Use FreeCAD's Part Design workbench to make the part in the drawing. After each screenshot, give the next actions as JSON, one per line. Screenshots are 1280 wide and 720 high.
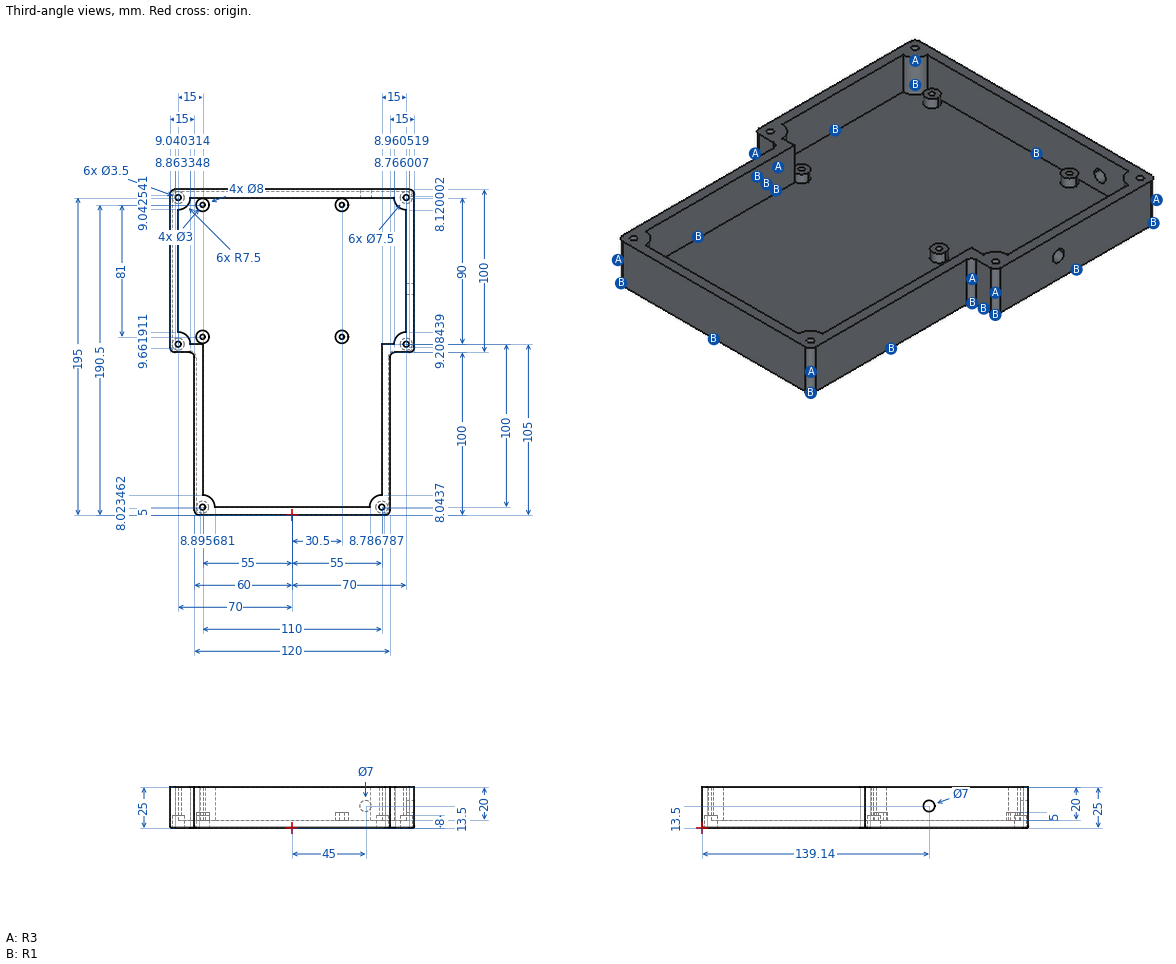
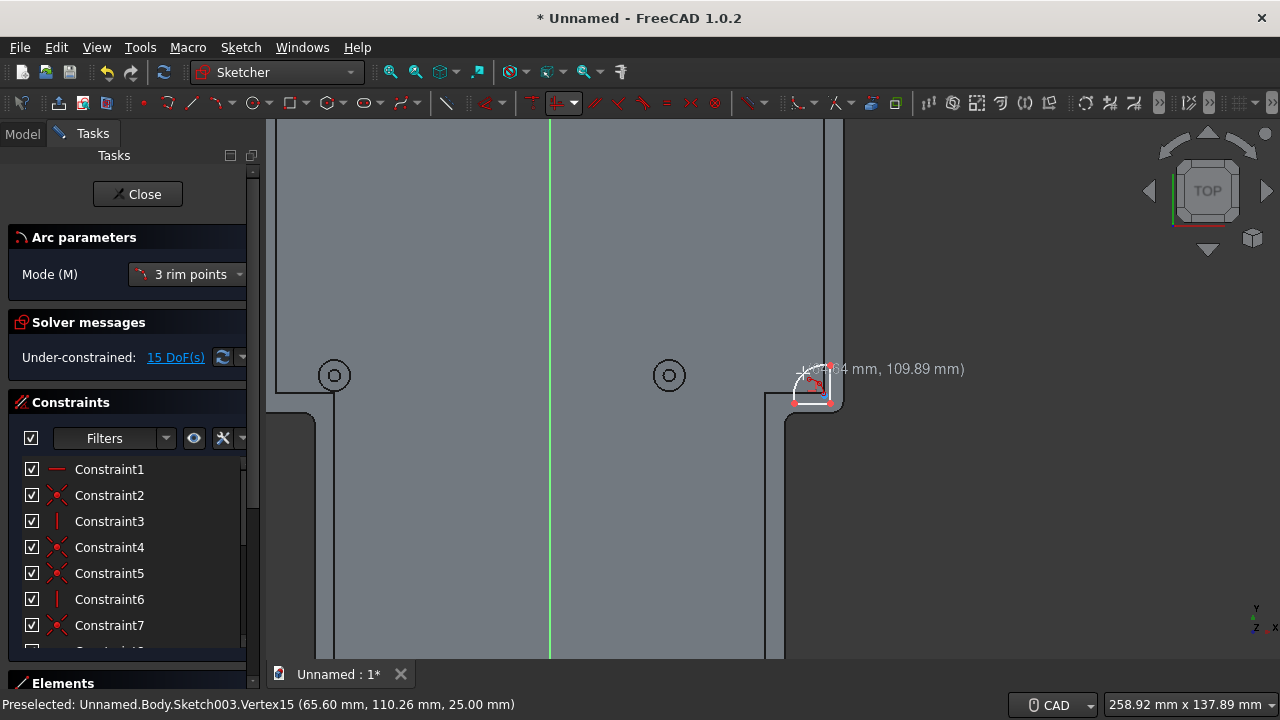
{"action": "key", "text": "g m"}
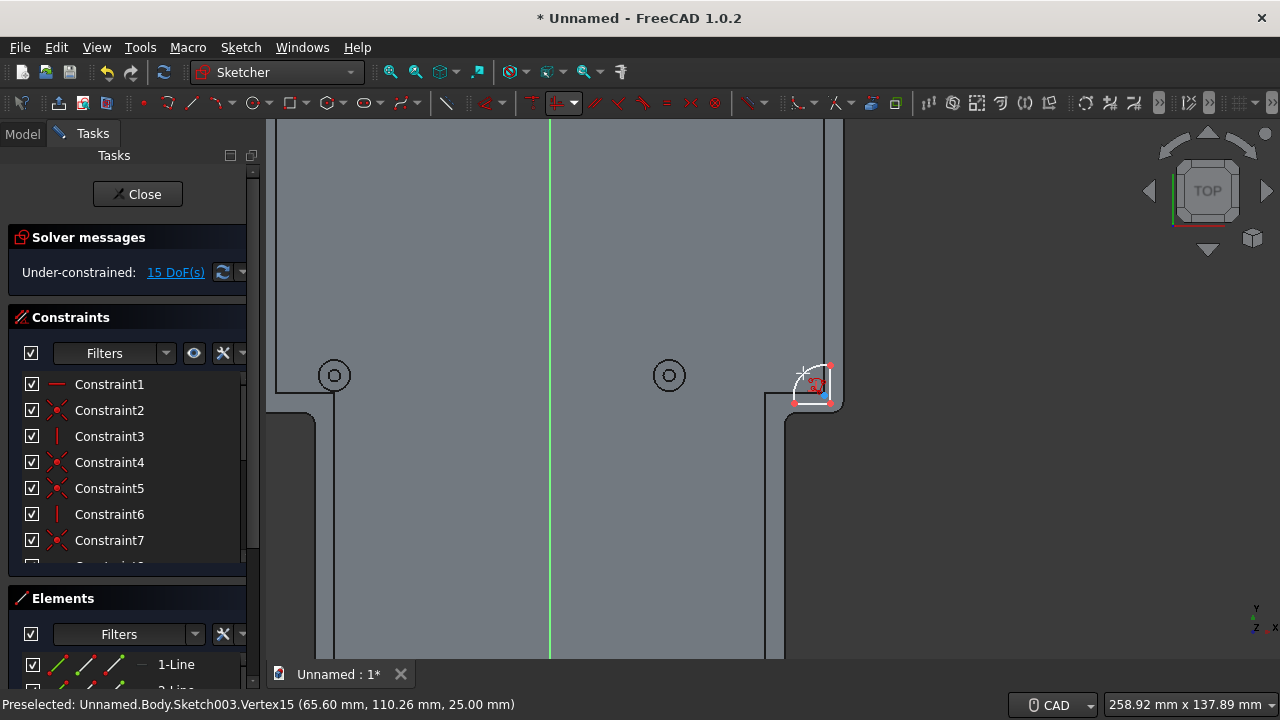
{"action": "scroll", "coordinate": [831, 364], "scroll_direction": "down", "scroll_amount": 4}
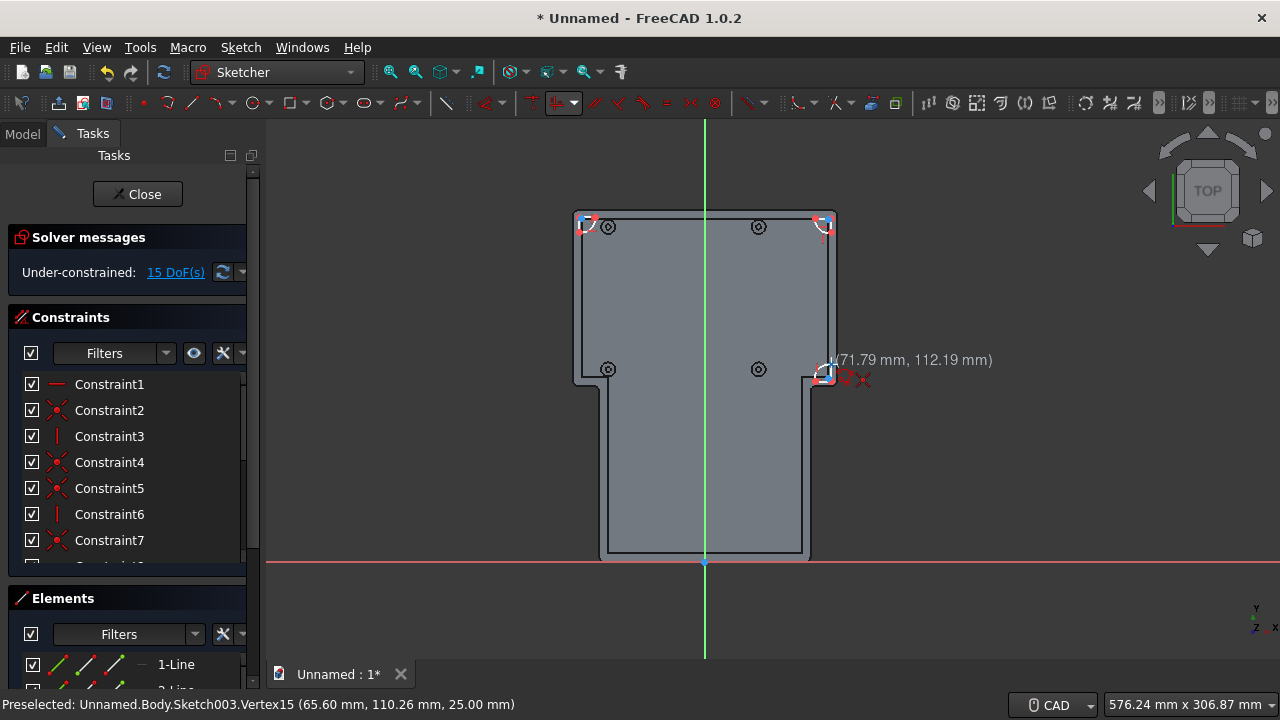
{"action": "left_click", "coordinate": [606, 540]}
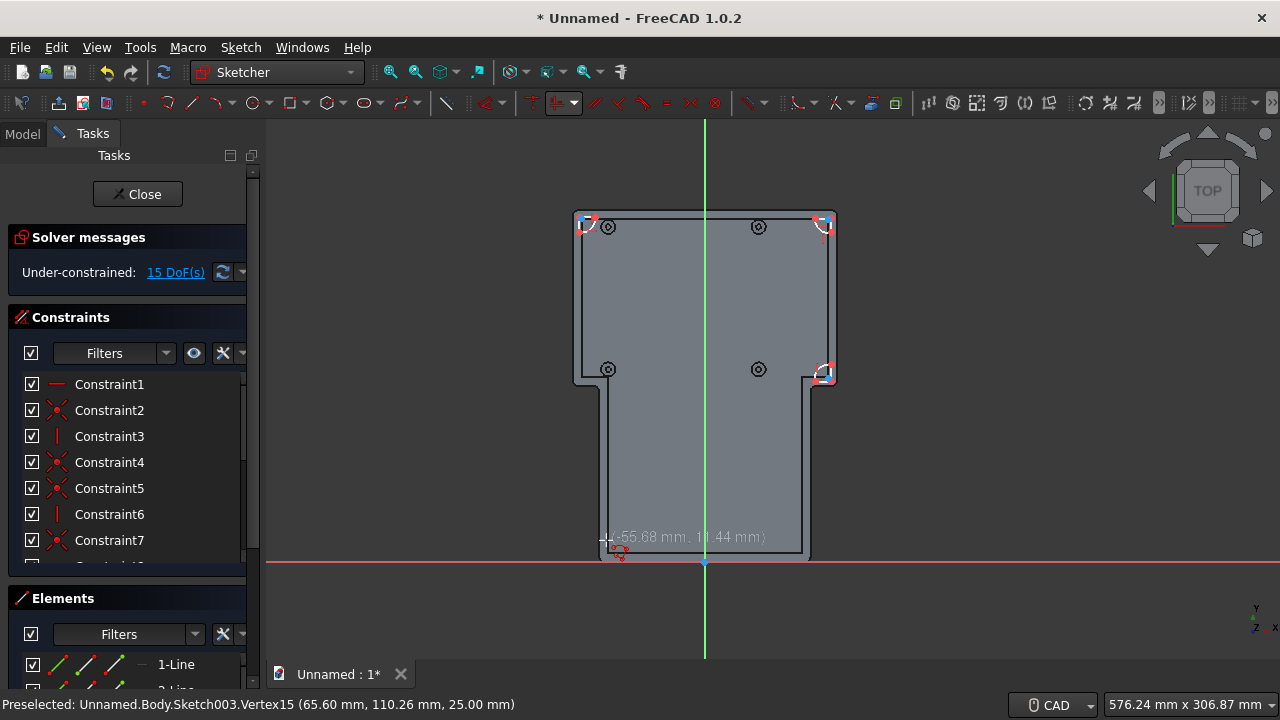
{"action": "scroll", "coordinate": [606, 554], "scroll_direction": "up", "scroll_amount": 4}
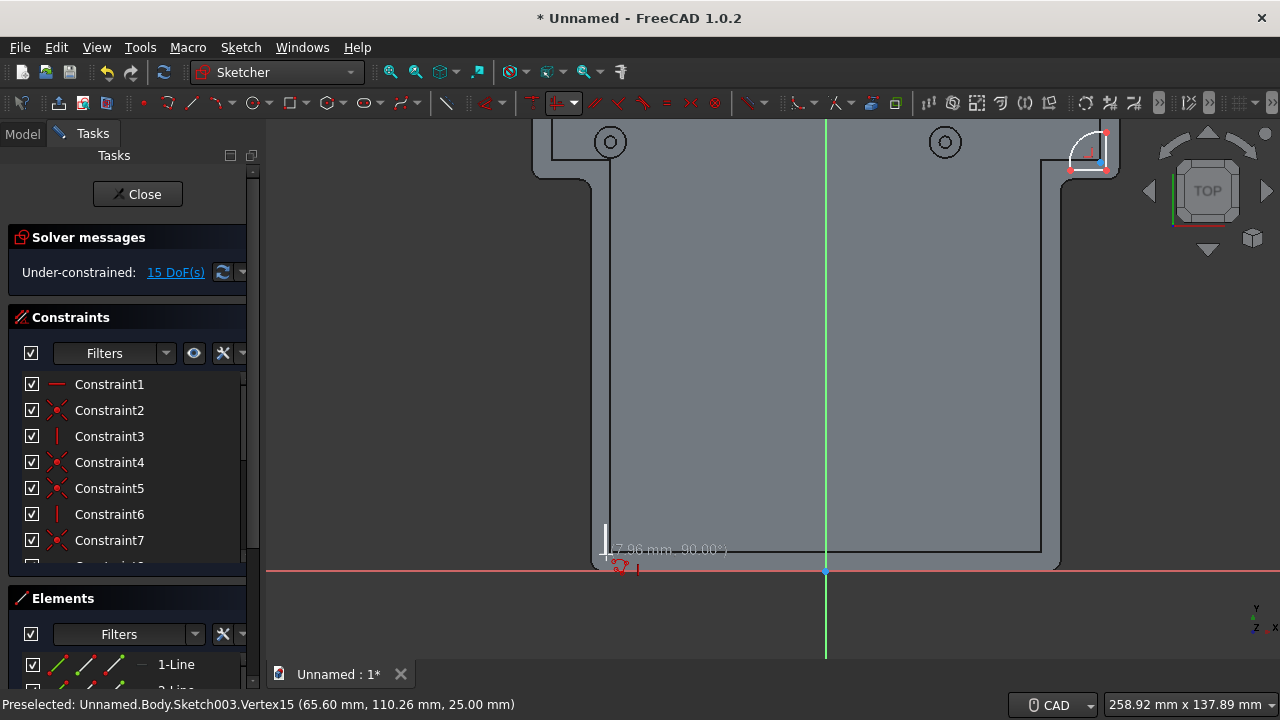
{"action": "left_click", "coordinate": [606, 554]}
{"action": "left_click", "coordinate": [640, 554]}
{"action": "right_click", "coordinate": [640, 554]}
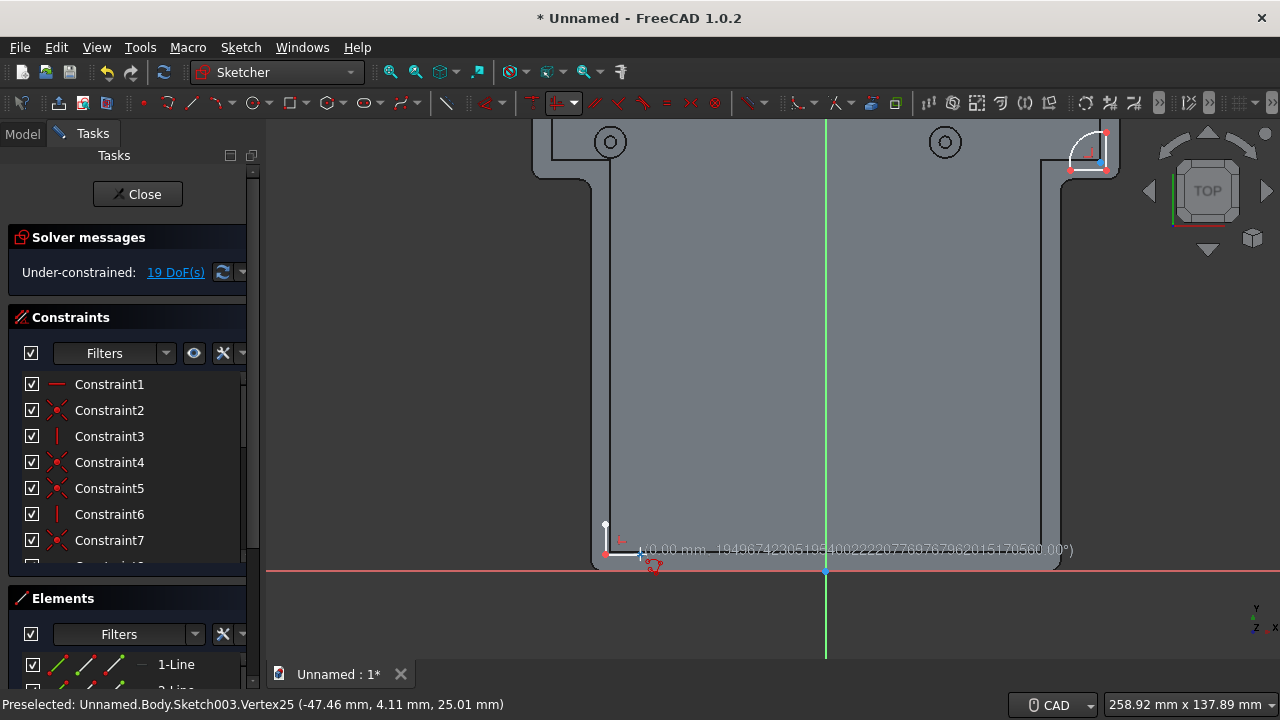
{"action": "key", "text": "g 3 a"}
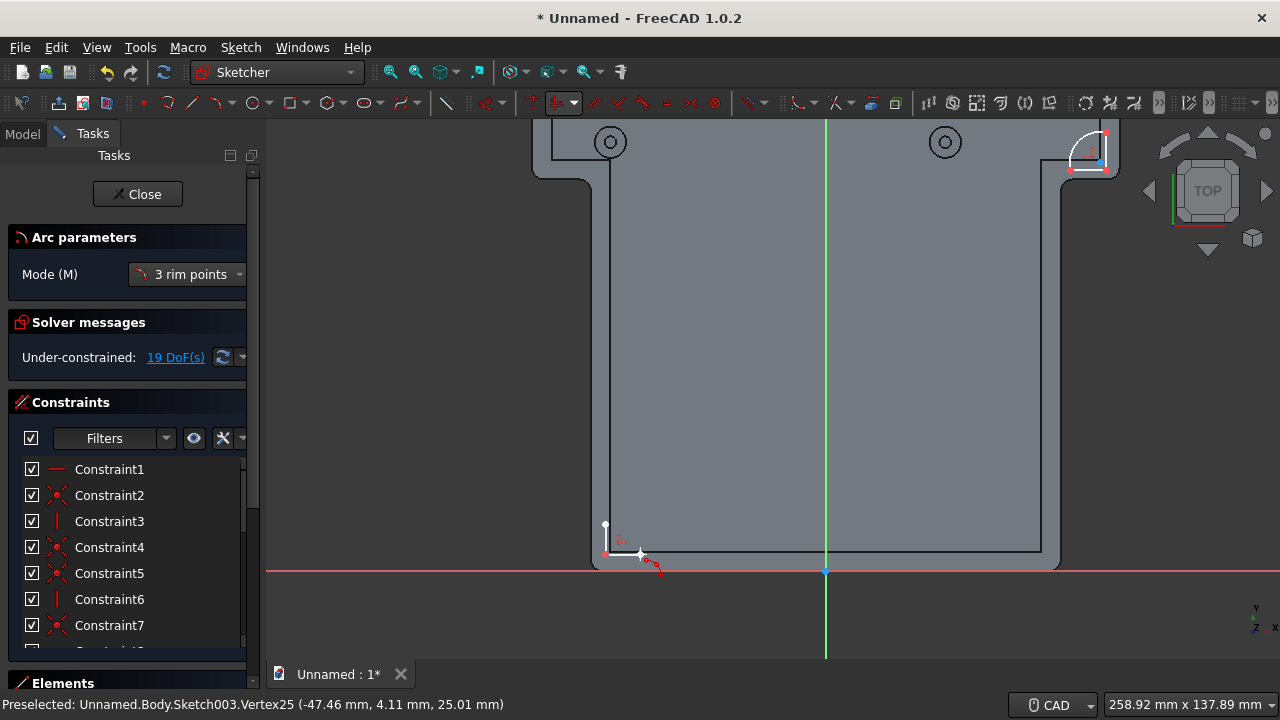
{"action": "left_click", "coordinate": [640, 555]}
{"action": "left_click", "coordinate": [606, 524]}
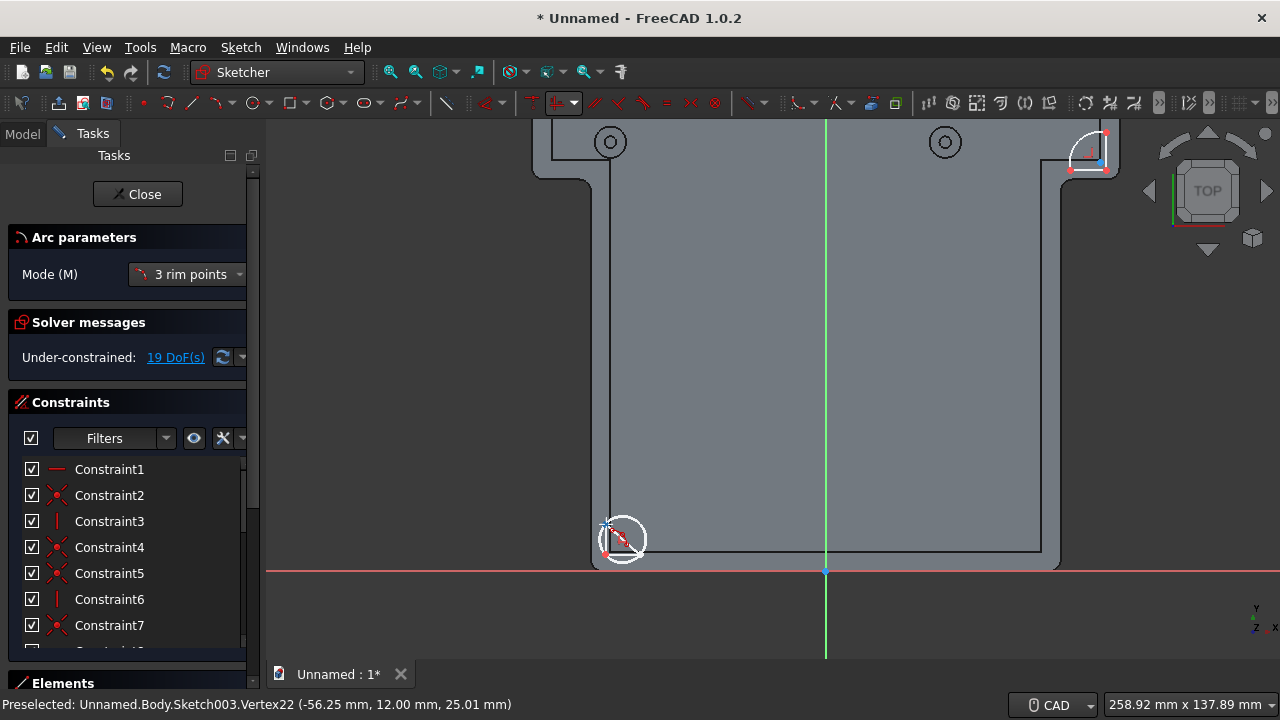
{"action": "scroll", "coordinate": [630, 530], "scroll_direction": "up", "scroll_amount": 2}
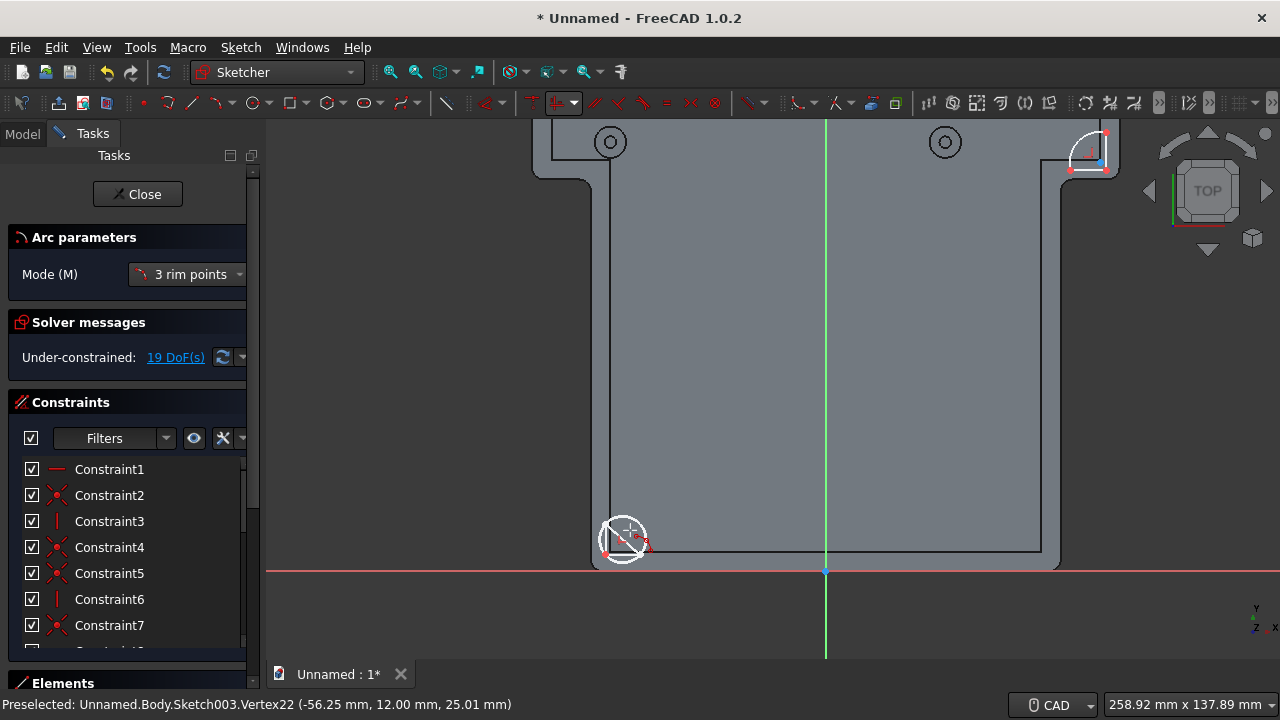
{"action": "left_click", "coordinate": [630, 529]}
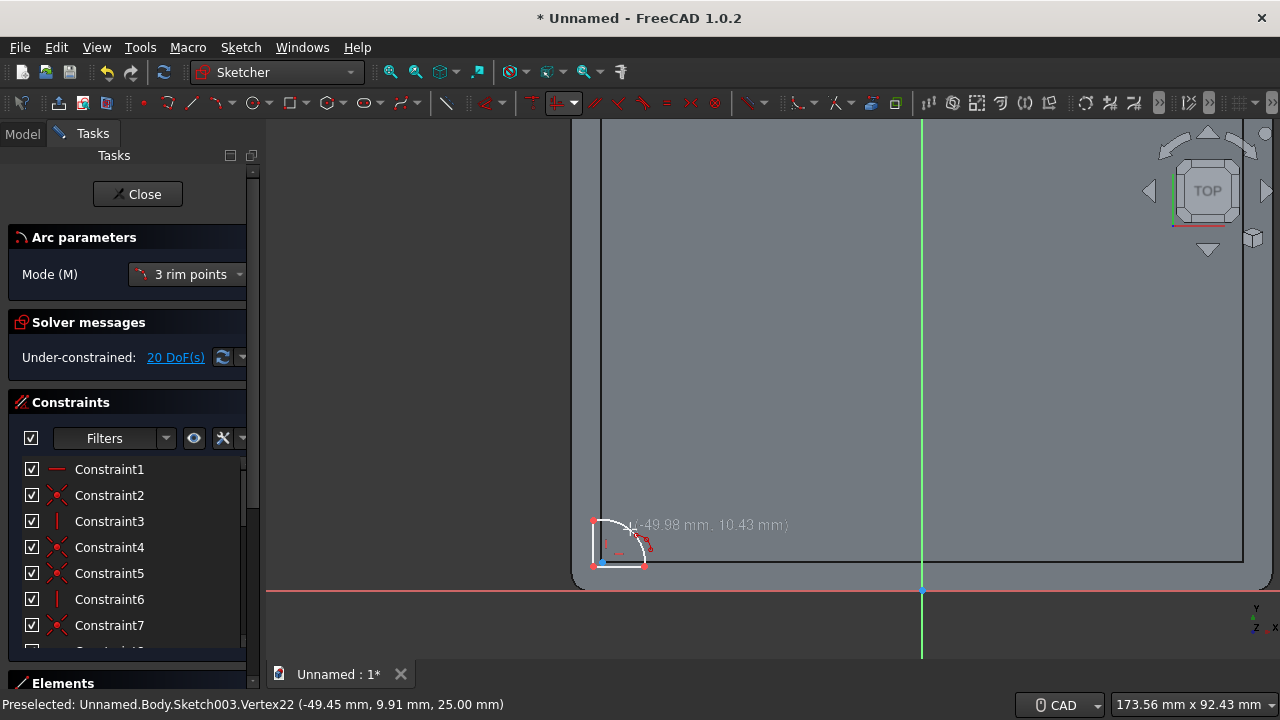
{"action": "key", "text": "g m"}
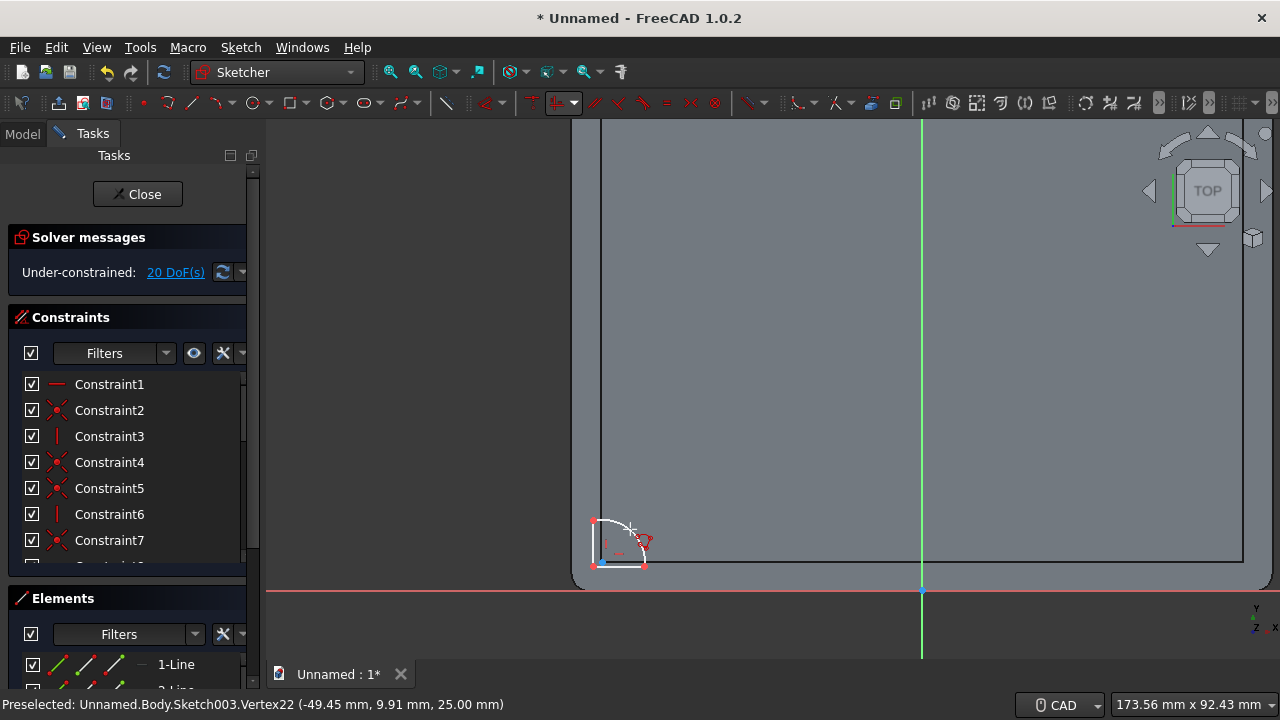
{"action": "scroll", "coordinate": [611, 550], "scroll_direction": "down", "scroll_amount": 6}